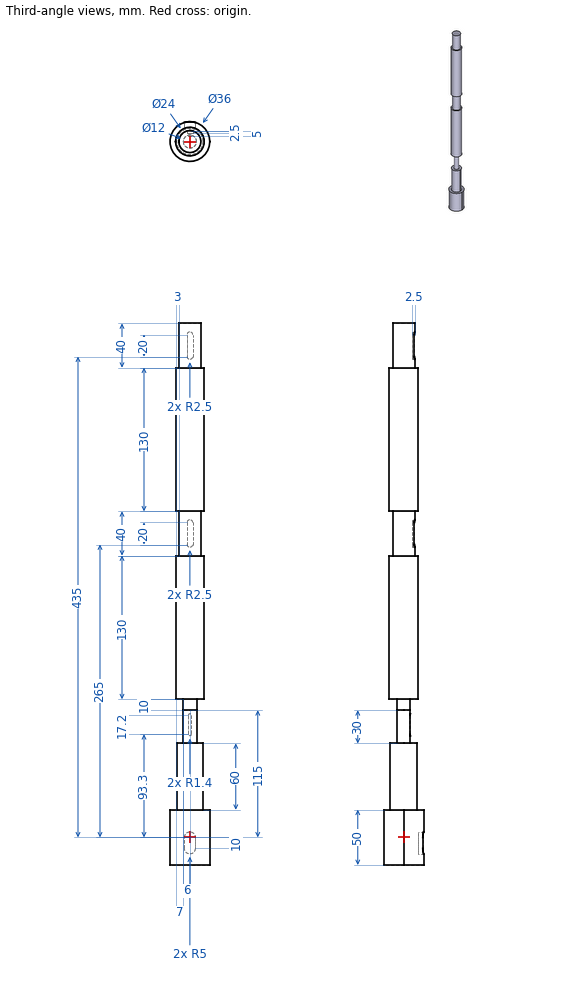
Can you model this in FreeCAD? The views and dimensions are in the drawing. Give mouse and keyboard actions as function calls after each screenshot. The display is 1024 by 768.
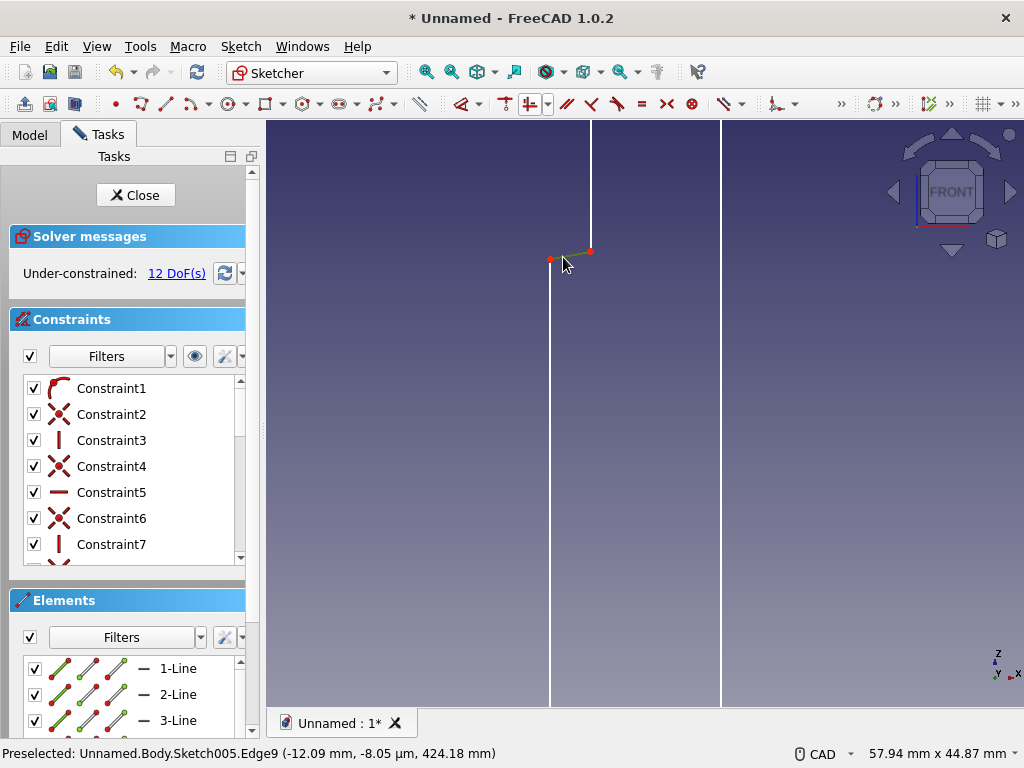
key(h)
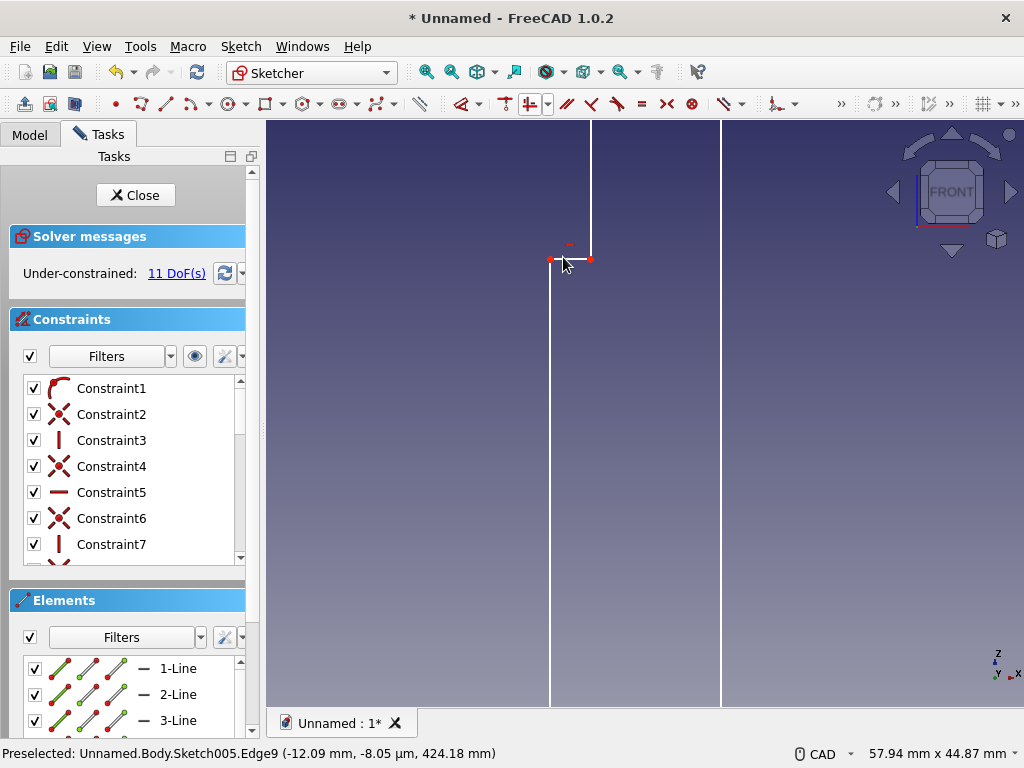
click(460, 104)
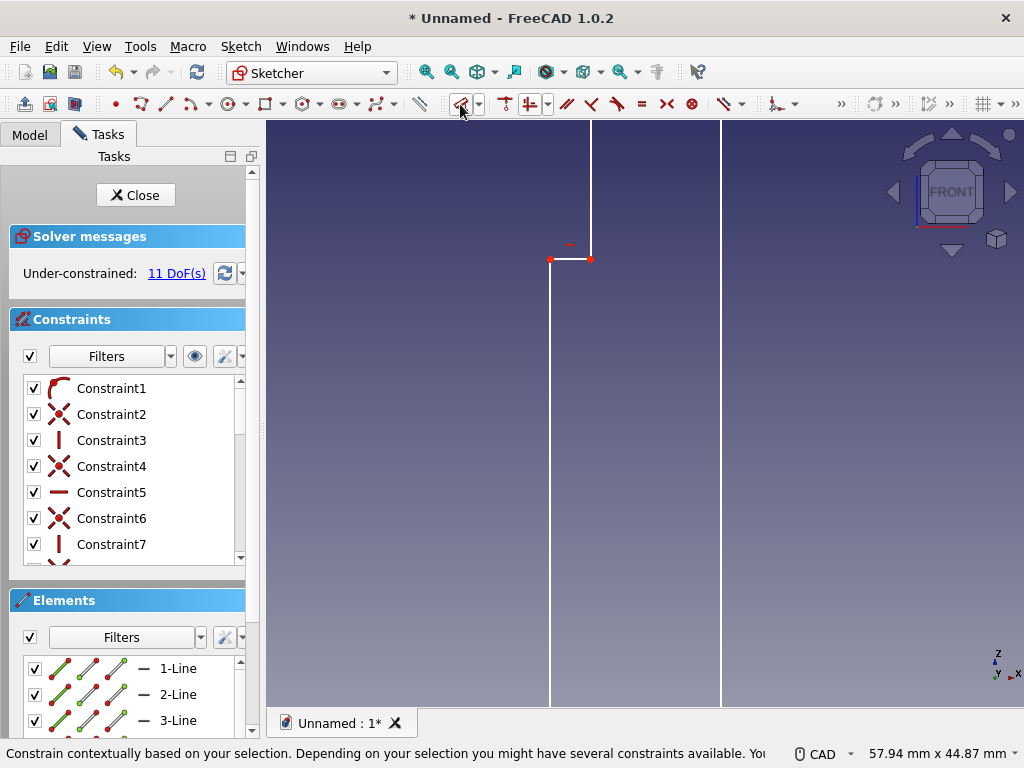
scroll(573, 261, down, 14)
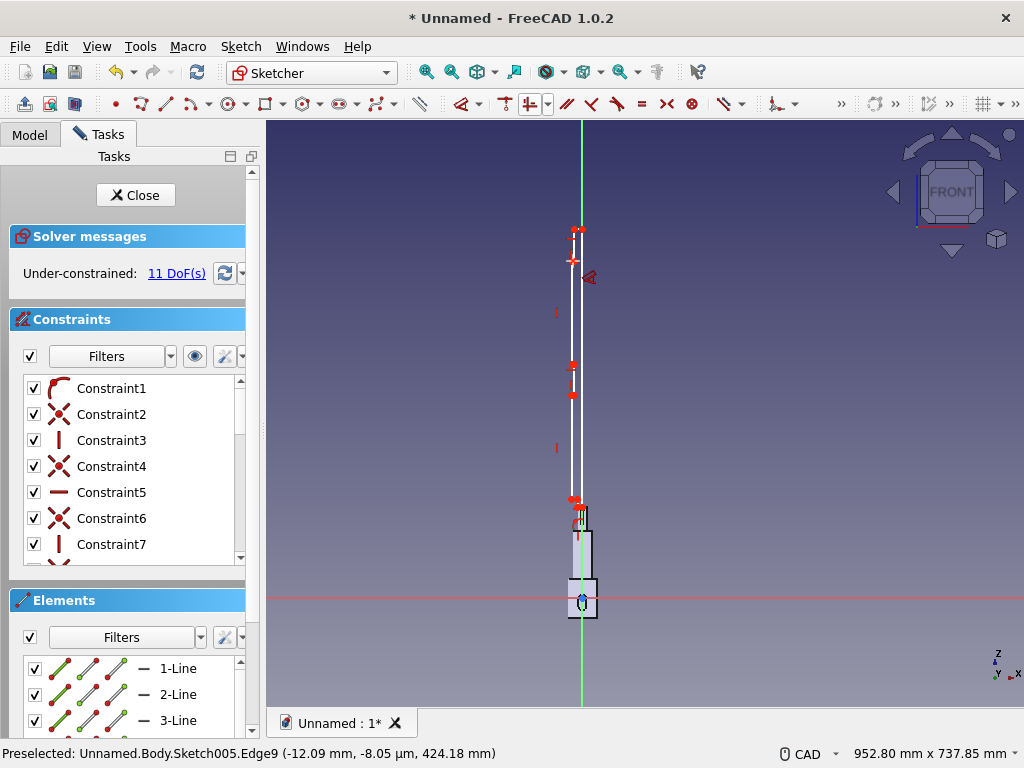
scroll(581, 508, up, 12)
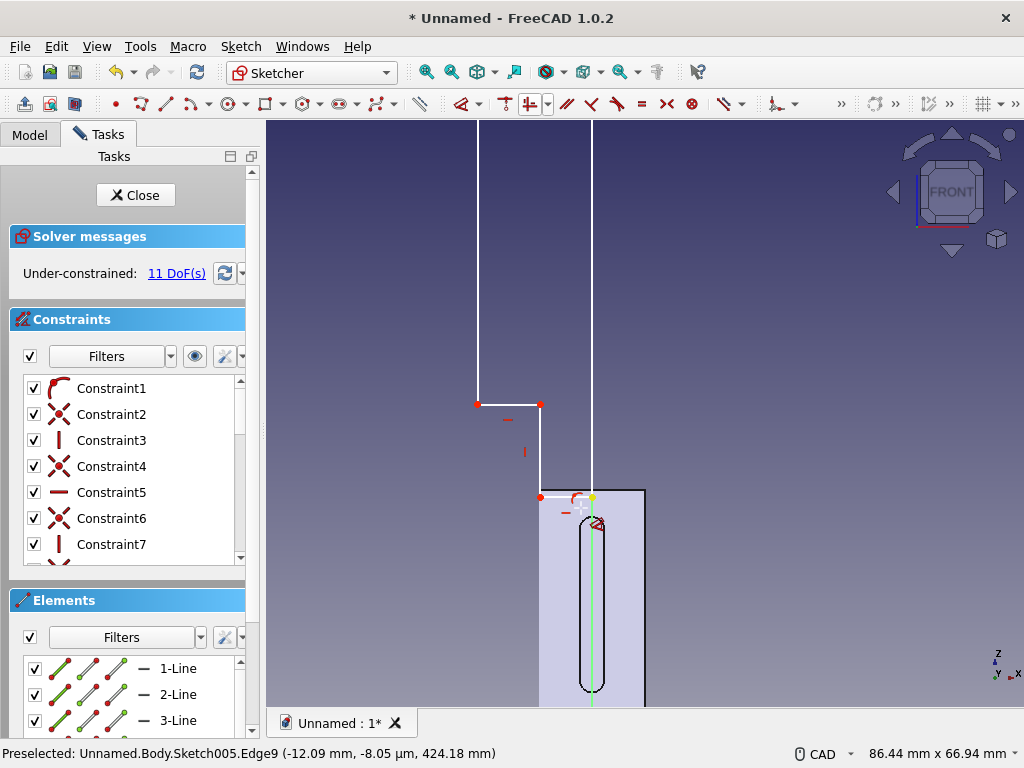
click(576, 497)
click(566, 531)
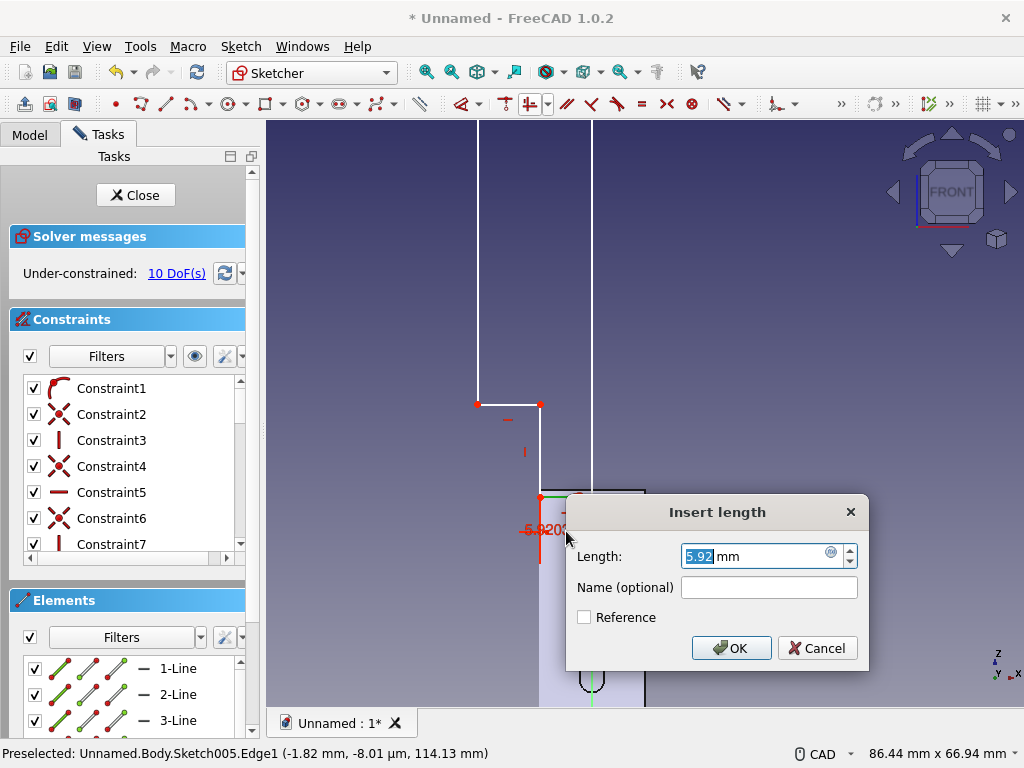
text(6)
key(Return)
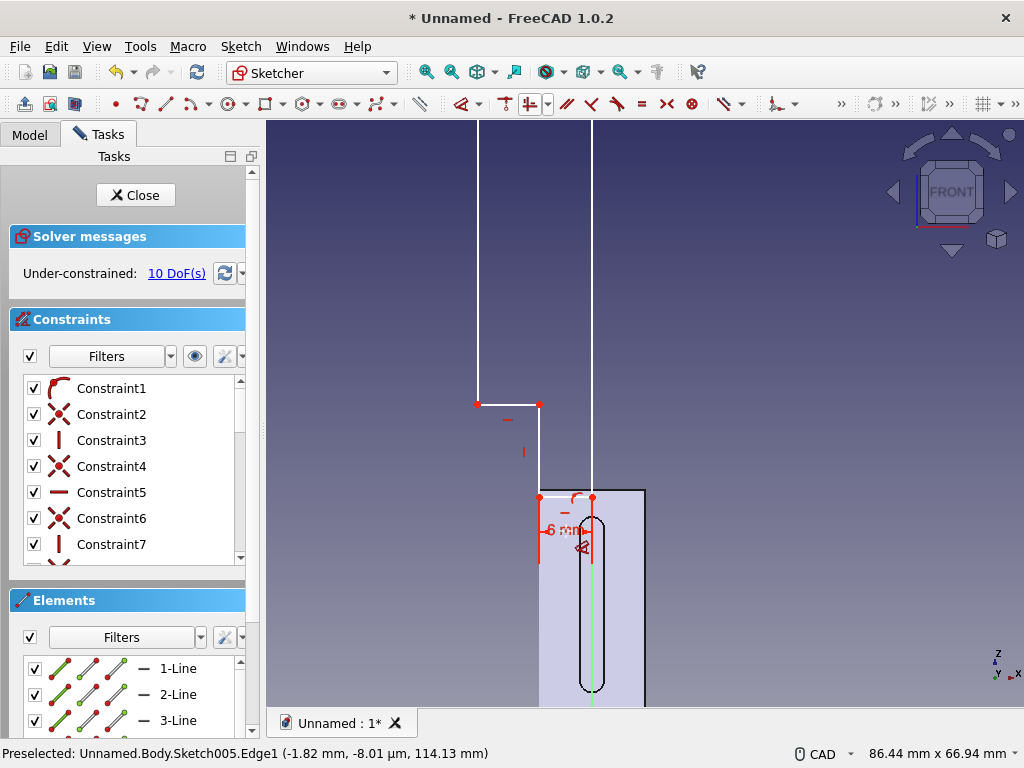
click(521, 405)
click(508, 439)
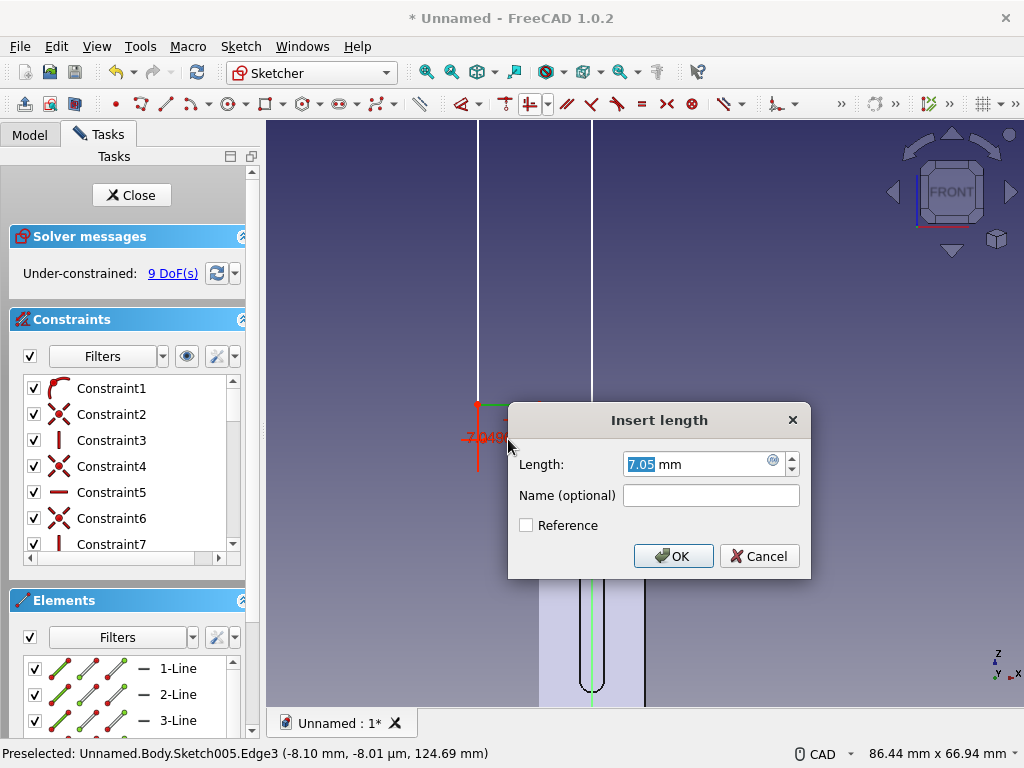
text(7)
key(Return)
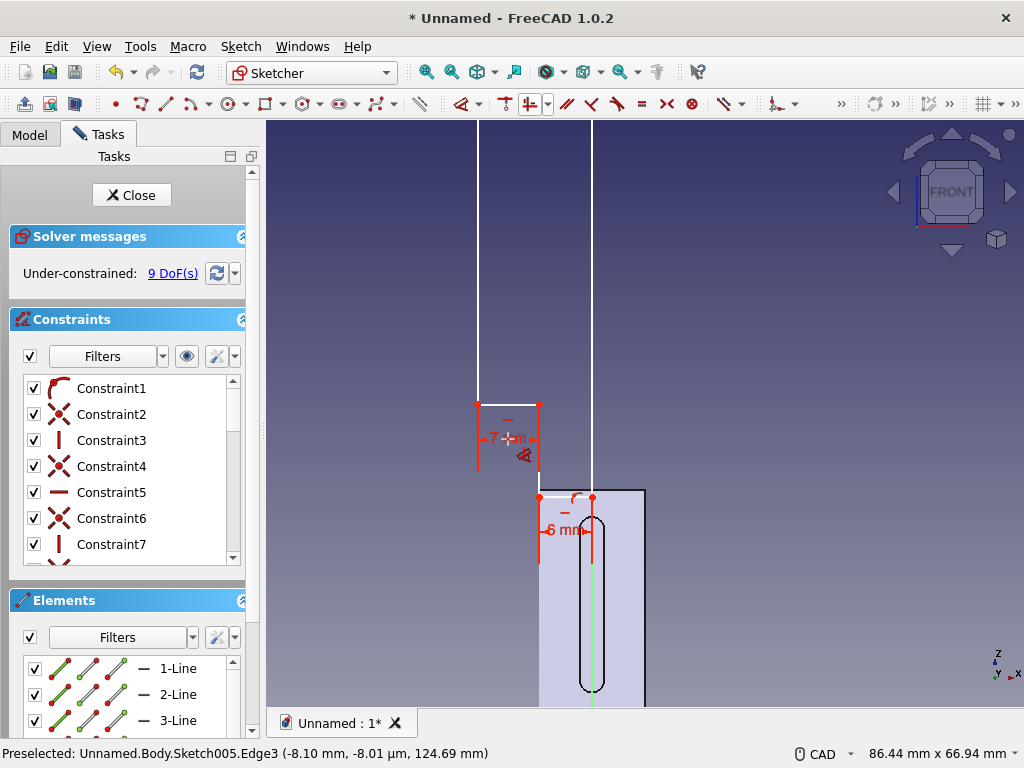
scroll(581, 509, down, 12)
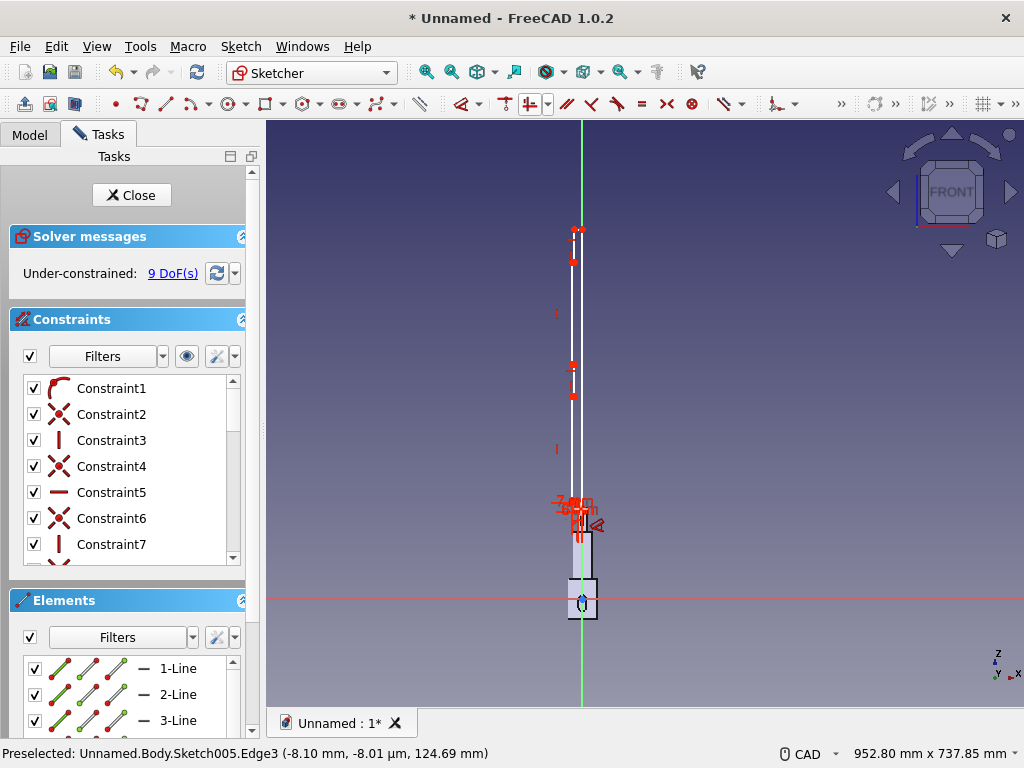
scroll(573, 397, up, 15)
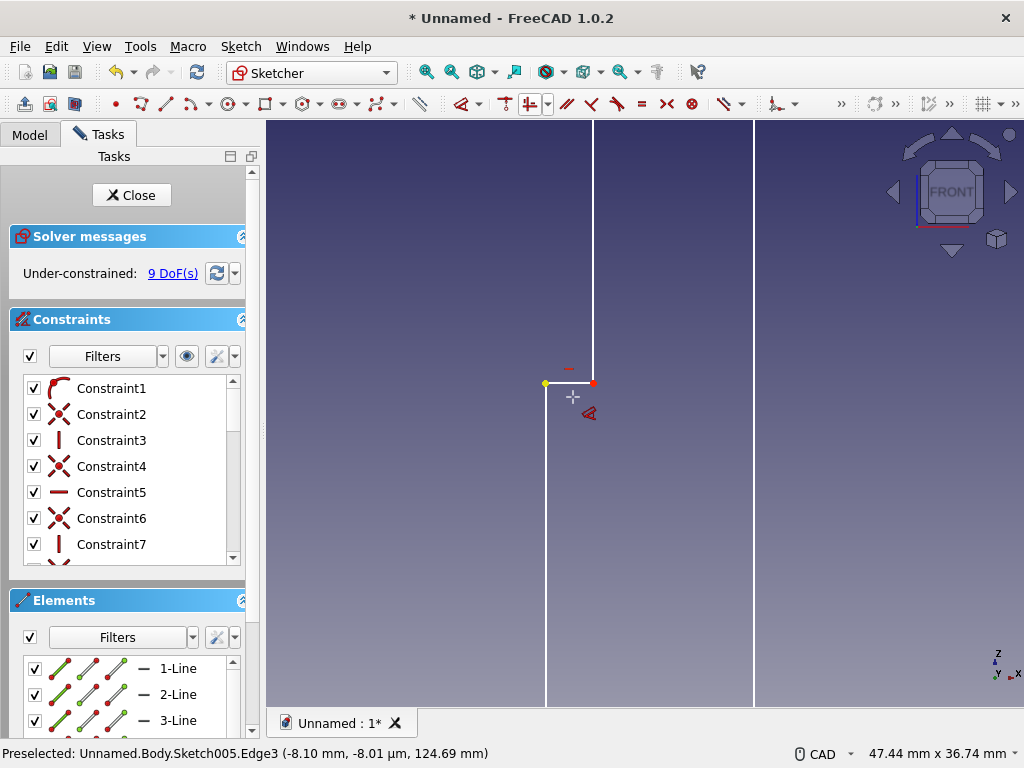
click(565, 383)
click(569, 349)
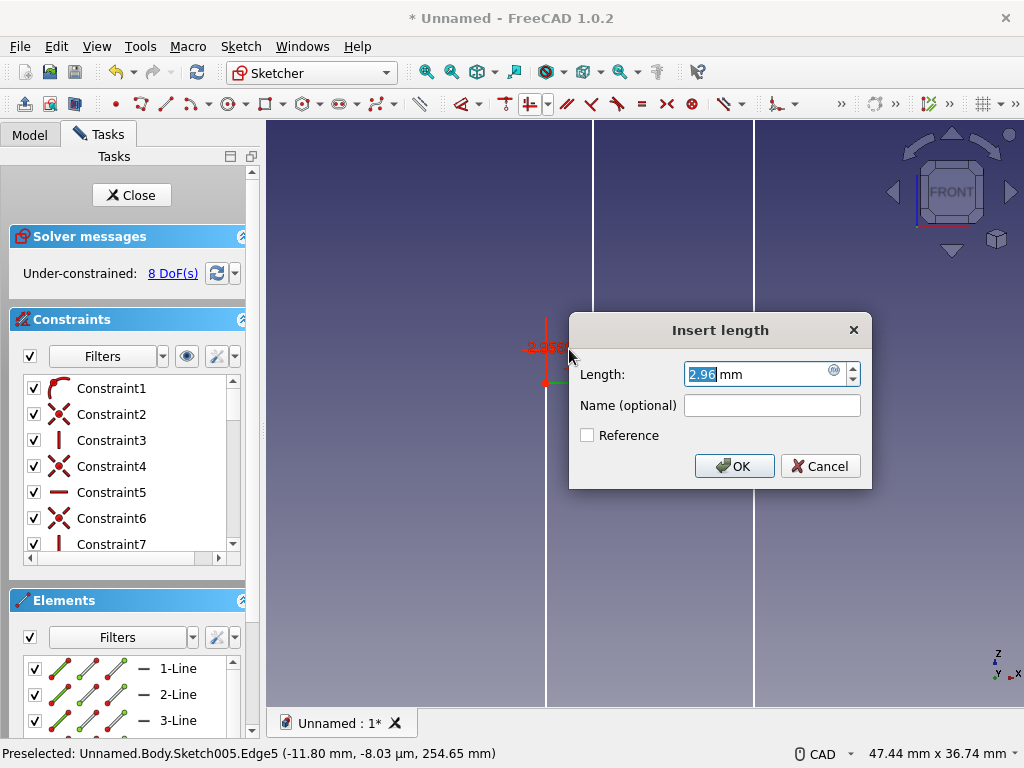
text(3)
key(Return)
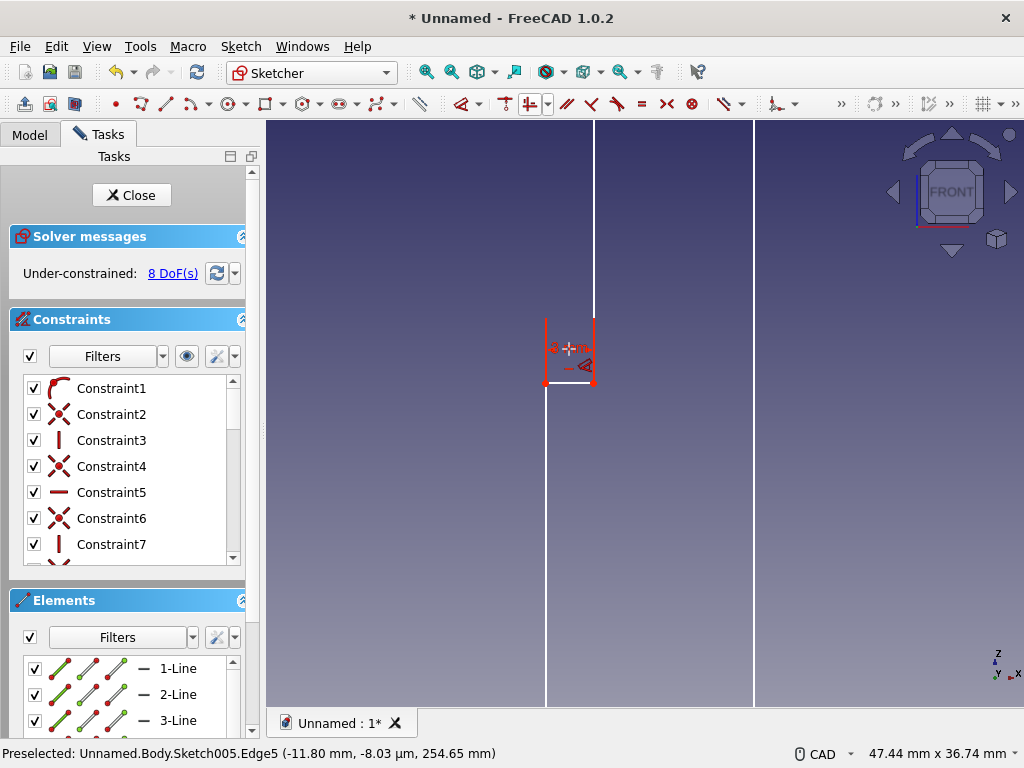
scroll(573, 397, down, 15)